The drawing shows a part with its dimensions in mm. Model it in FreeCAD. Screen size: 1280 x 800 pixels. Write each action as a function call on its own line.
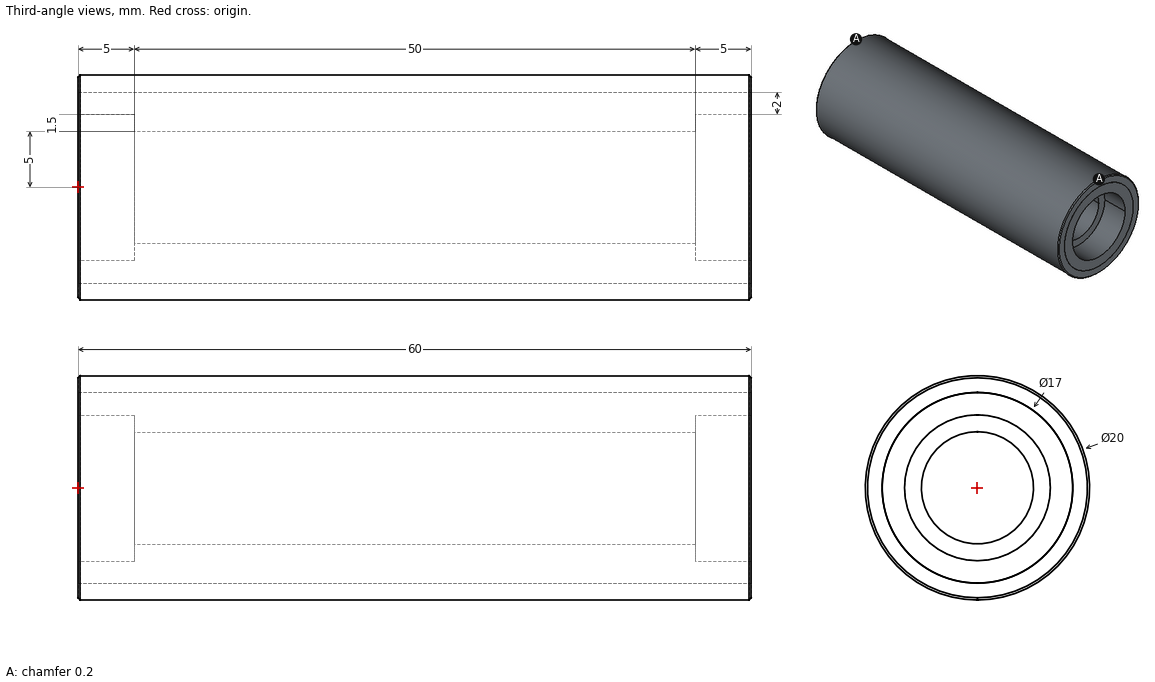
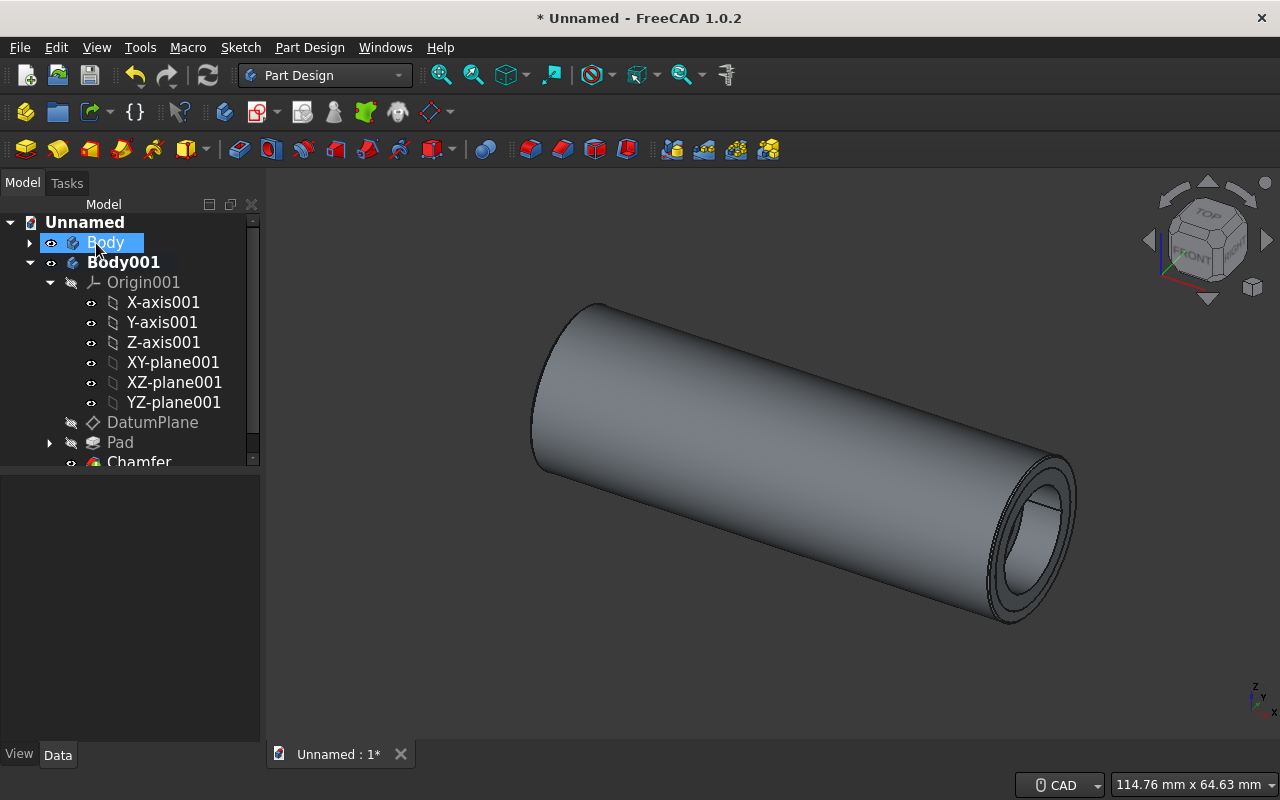
key(0)